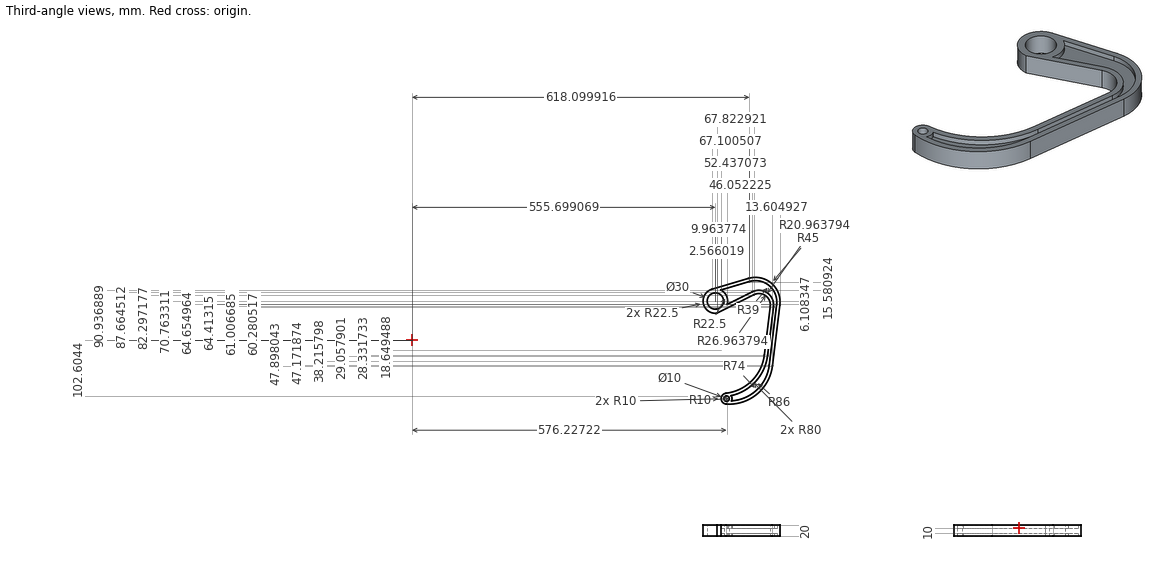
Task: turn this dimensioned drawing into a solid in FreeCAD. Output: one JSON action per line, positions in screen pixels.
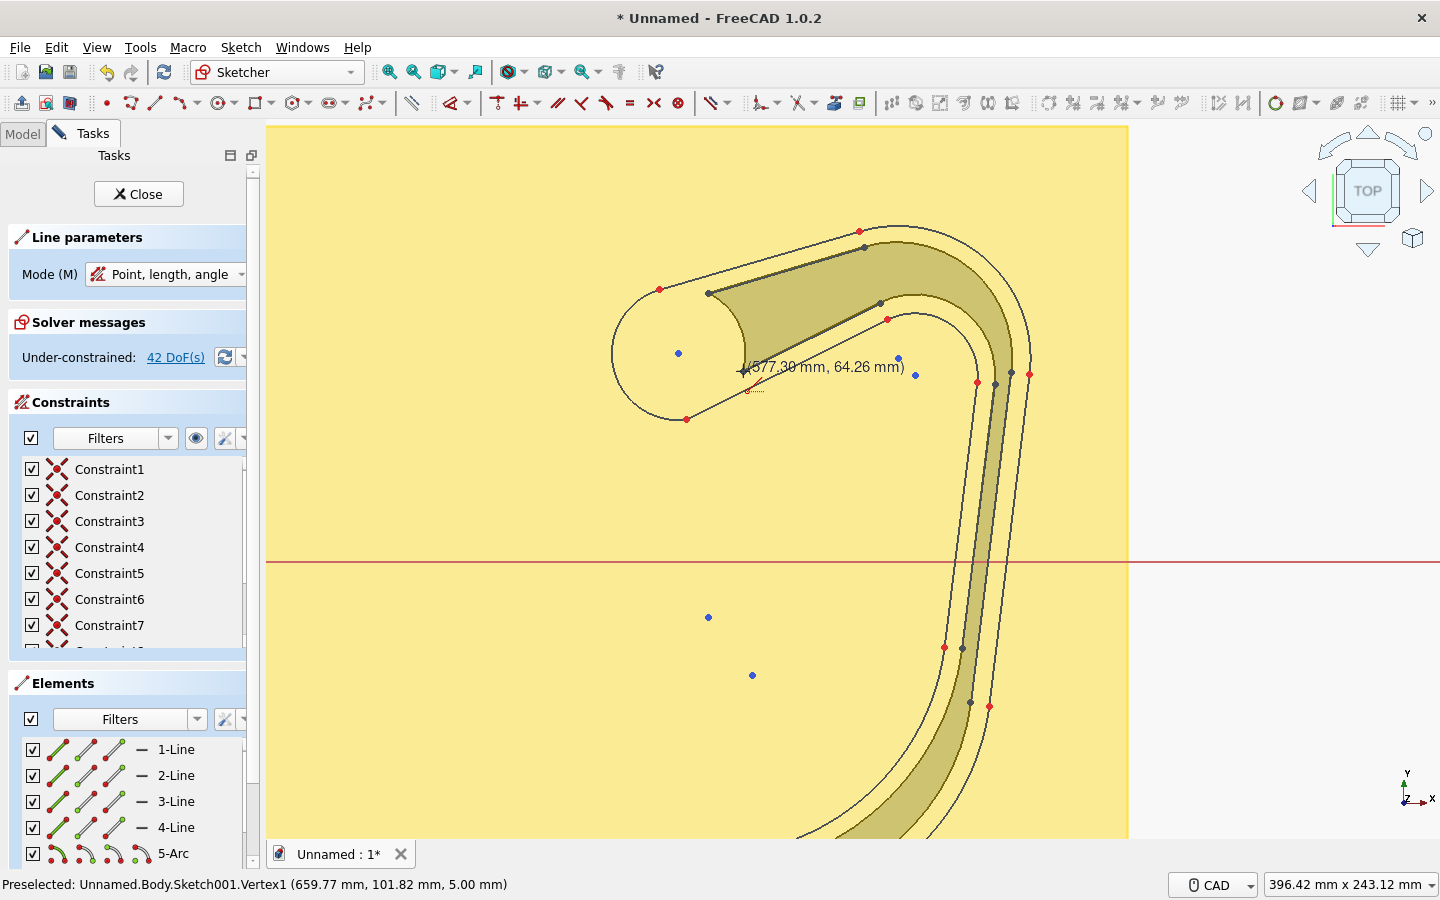
{"action": "left_click", "coordinate": [180, 104]}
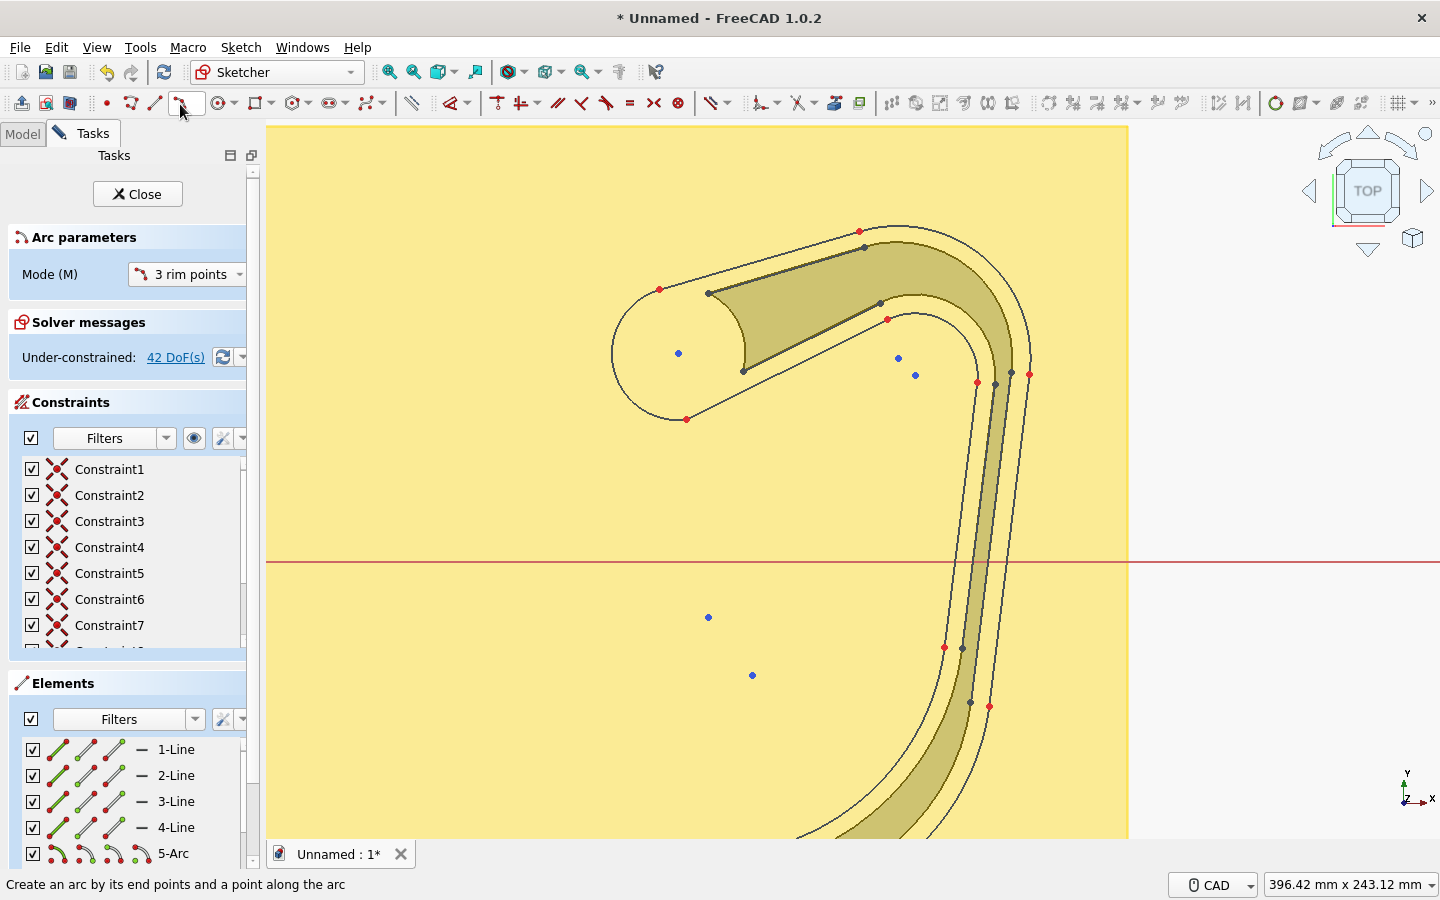
{"action": "left_click", "coordinate": [864, 248]}
{"action": "left_click", "coordinate": [1011, 373]}
{"action": "left_click", "coordinate": [1000, 305]}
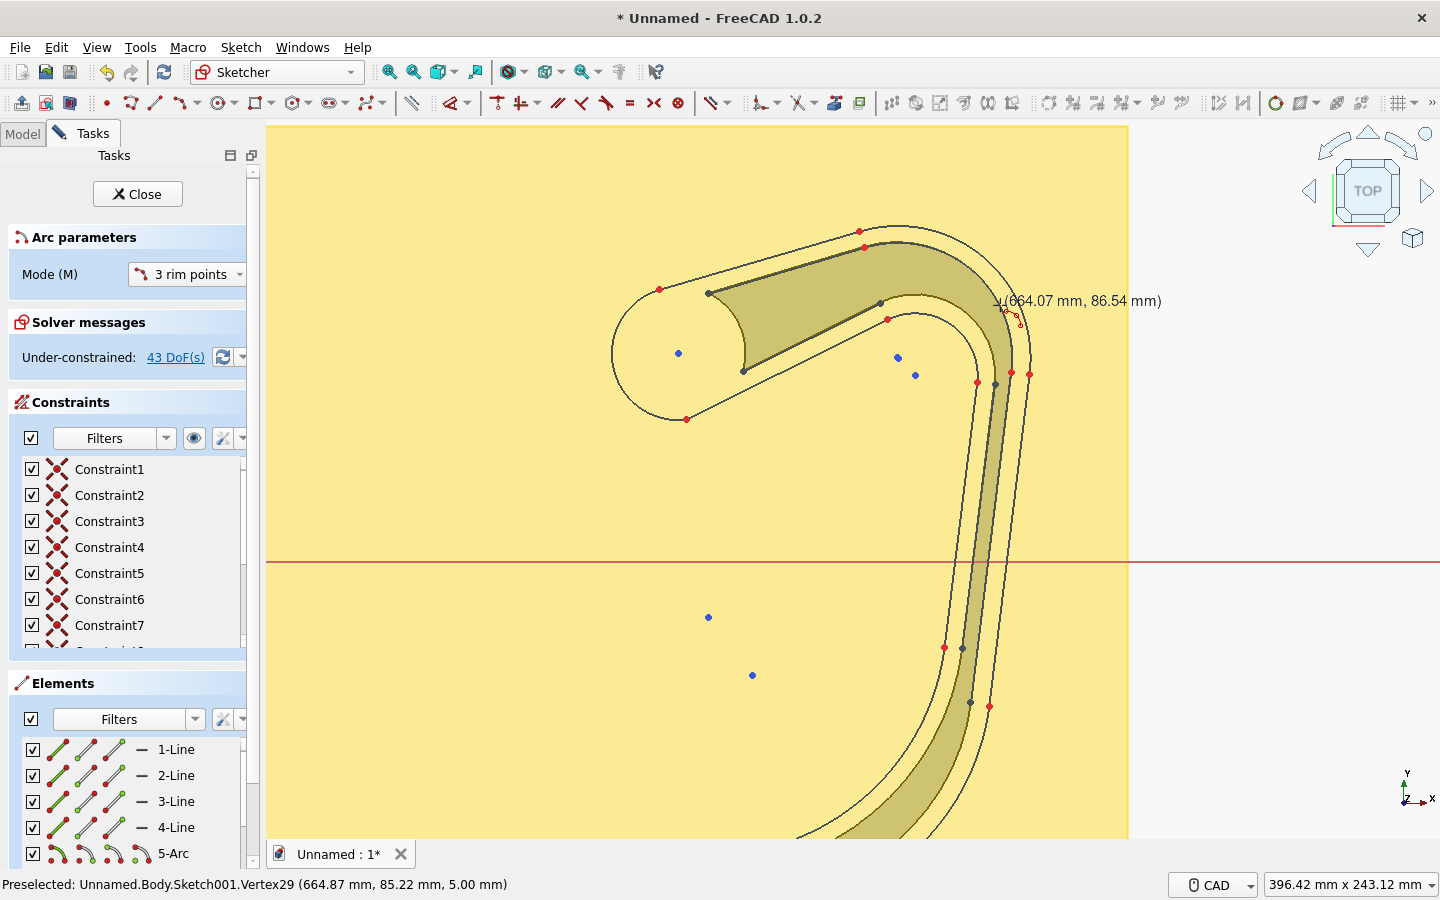
{"action": "left_click", "coordinate": [971, 703]}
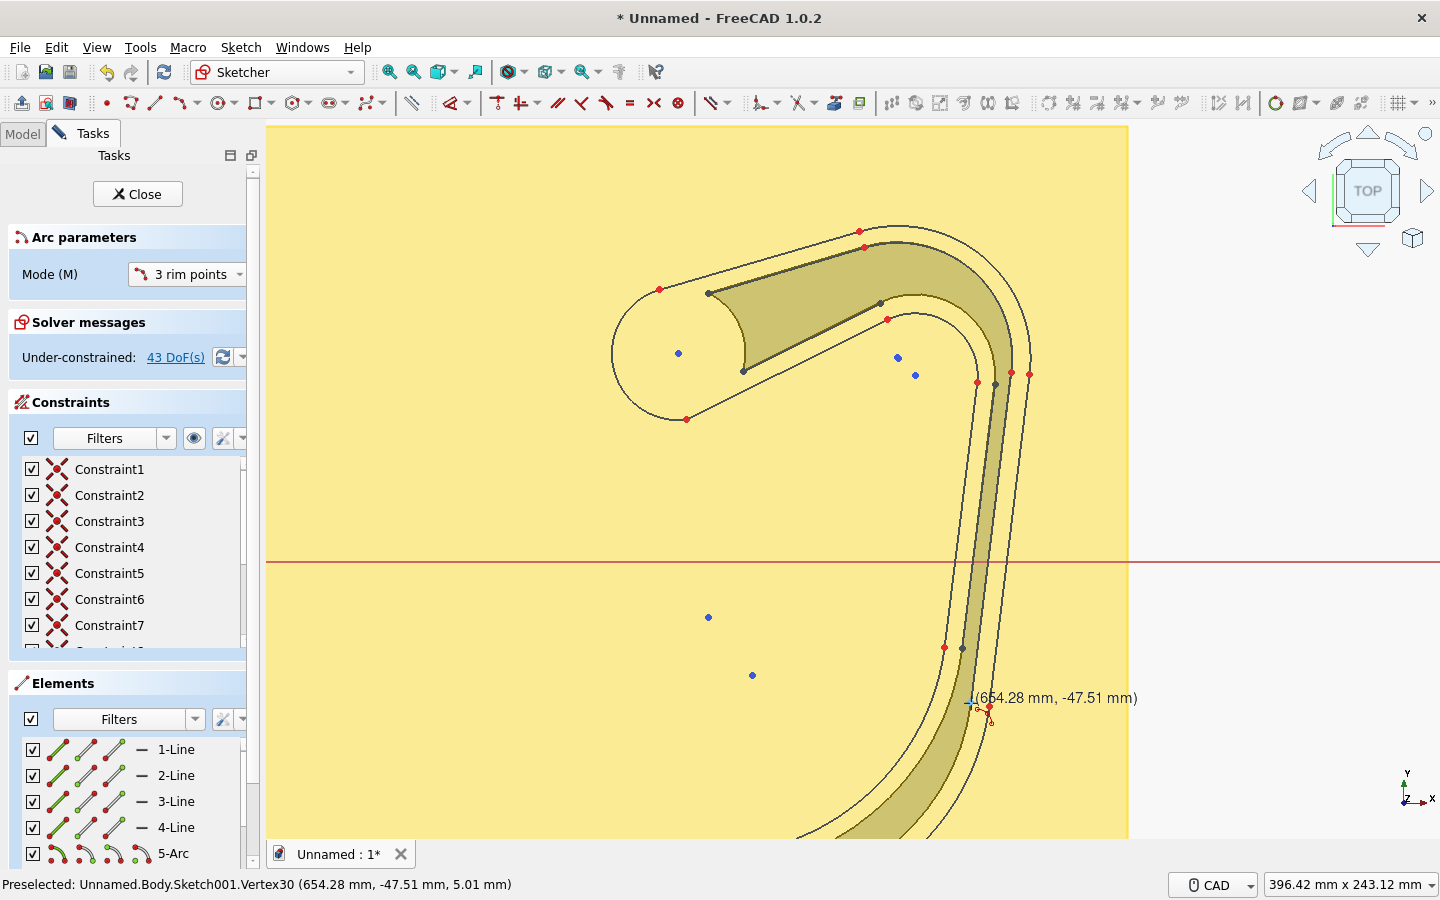
{"action": "scroll", "coordinate": [709, 292], "scroll_direction": "down", "scroll_amount": 2}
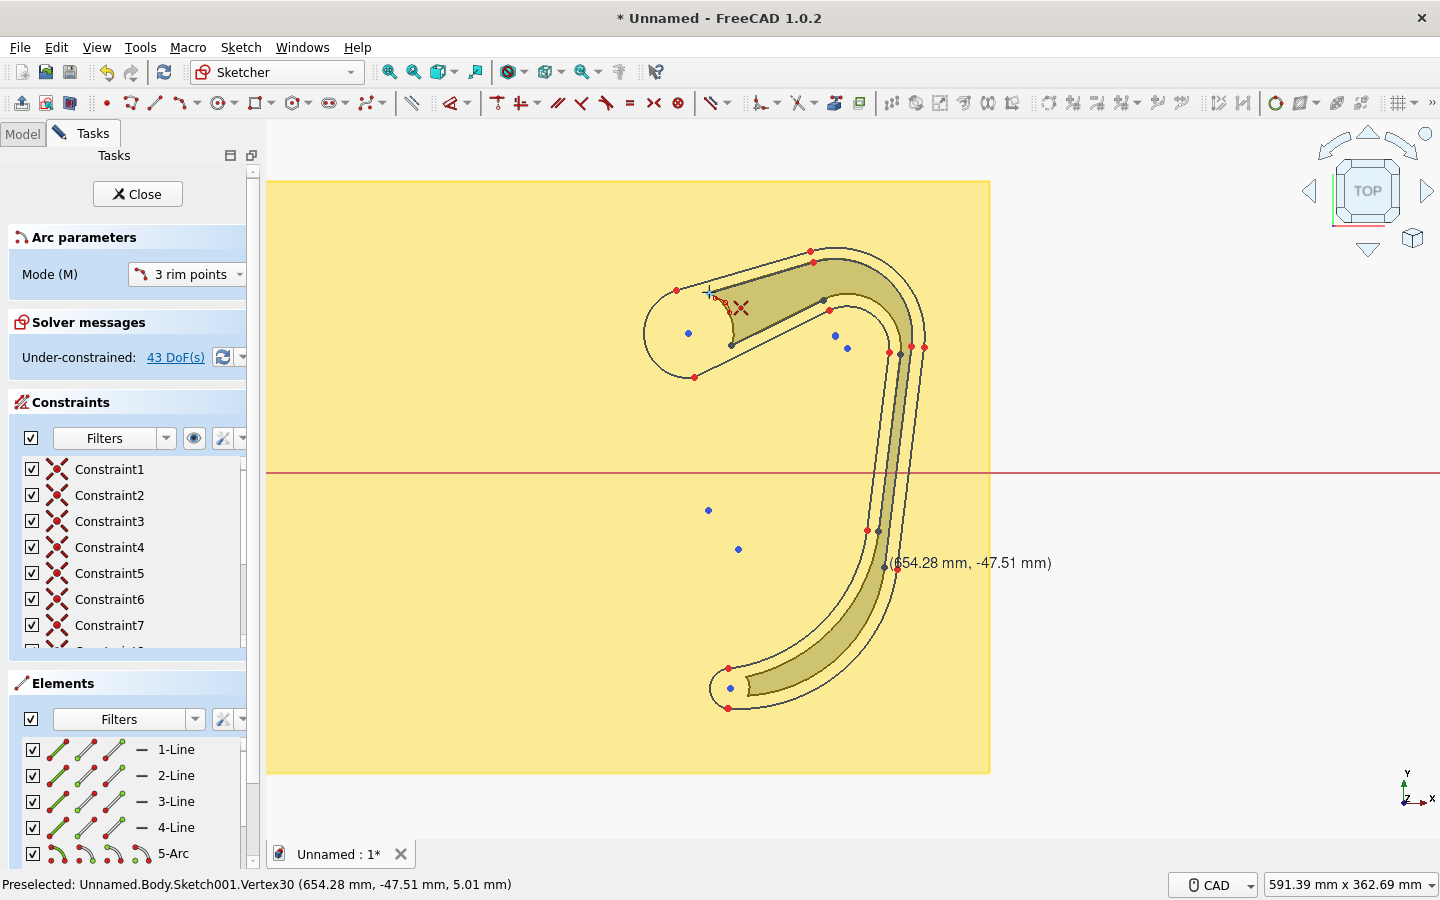
{"action": "scroll", "coordinate": [748, 696], "scroll_direction": "up", "scroll_amount": 2}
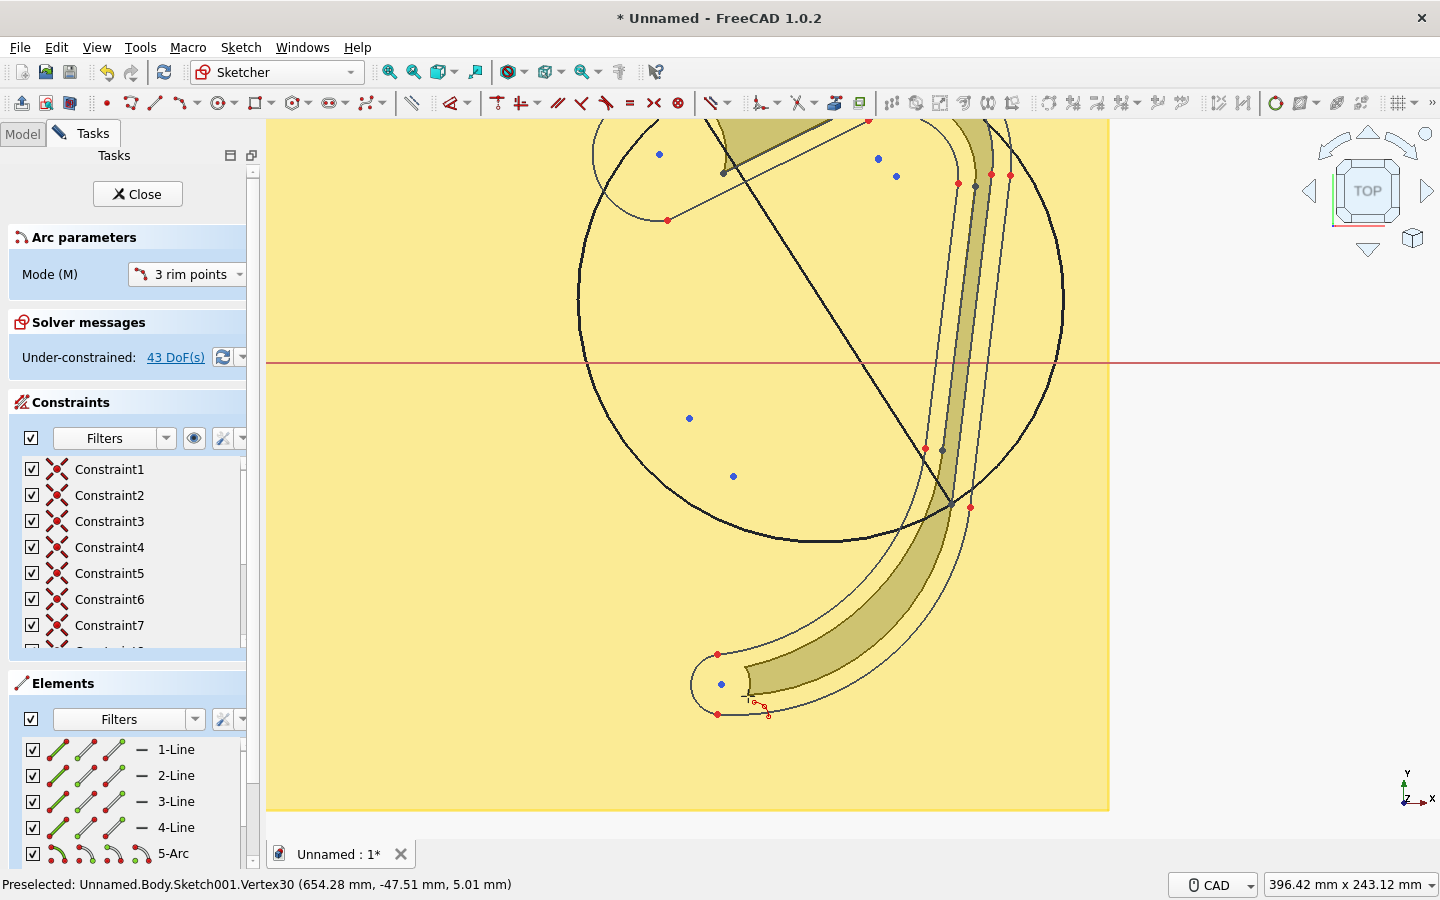
{"action": "left_click", "coordinate": [748, 695]}
{"action": "left_click", "coordinate": [861, 655]}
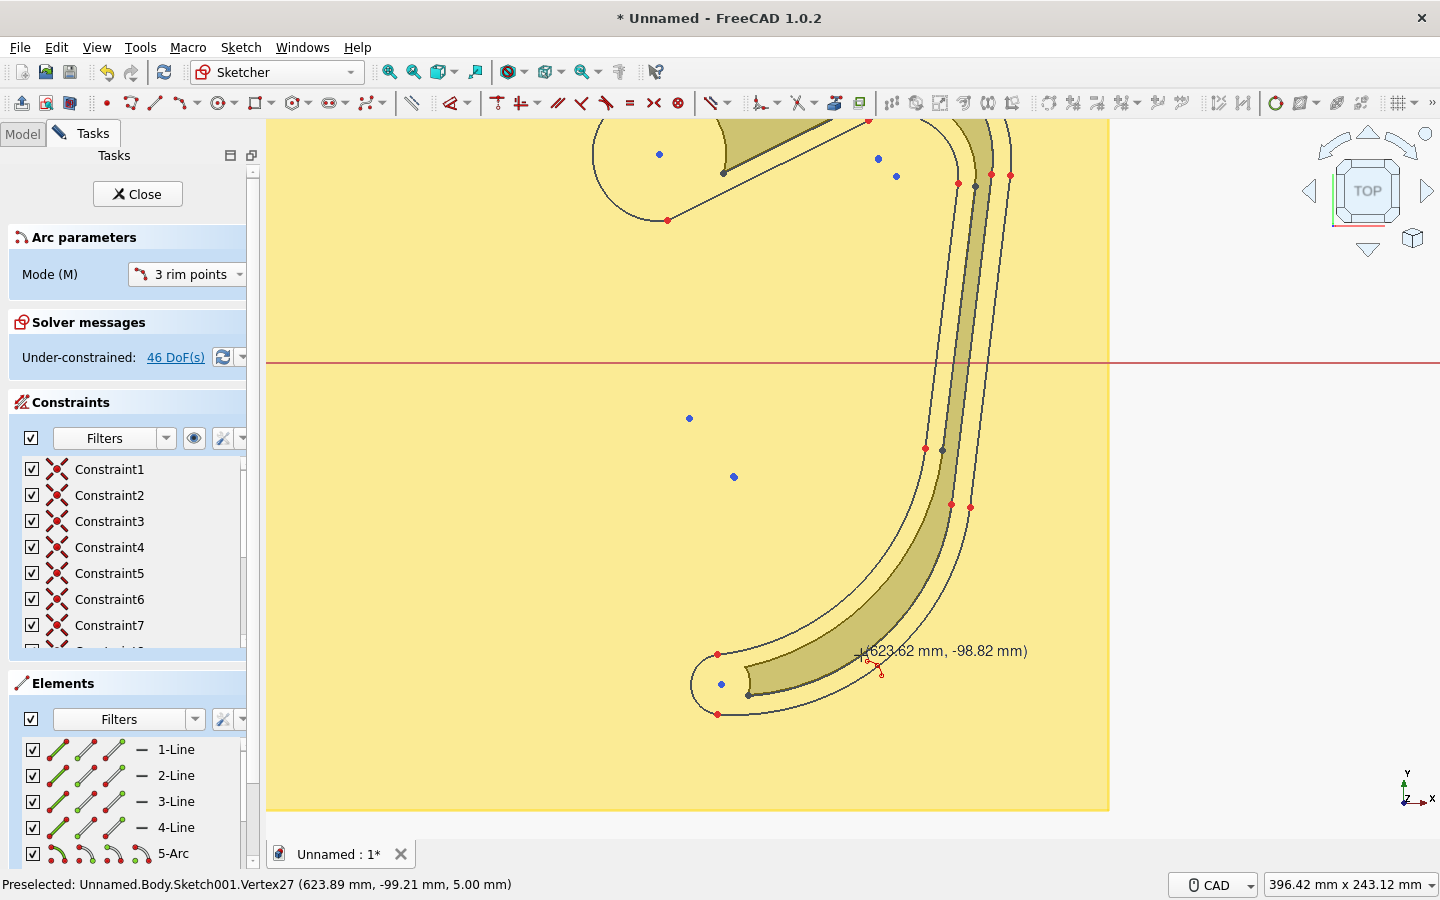
{"action": "left_click", "coordinate": [748, 696]}
{"action": "left_click", "coordinate": [745, 667]}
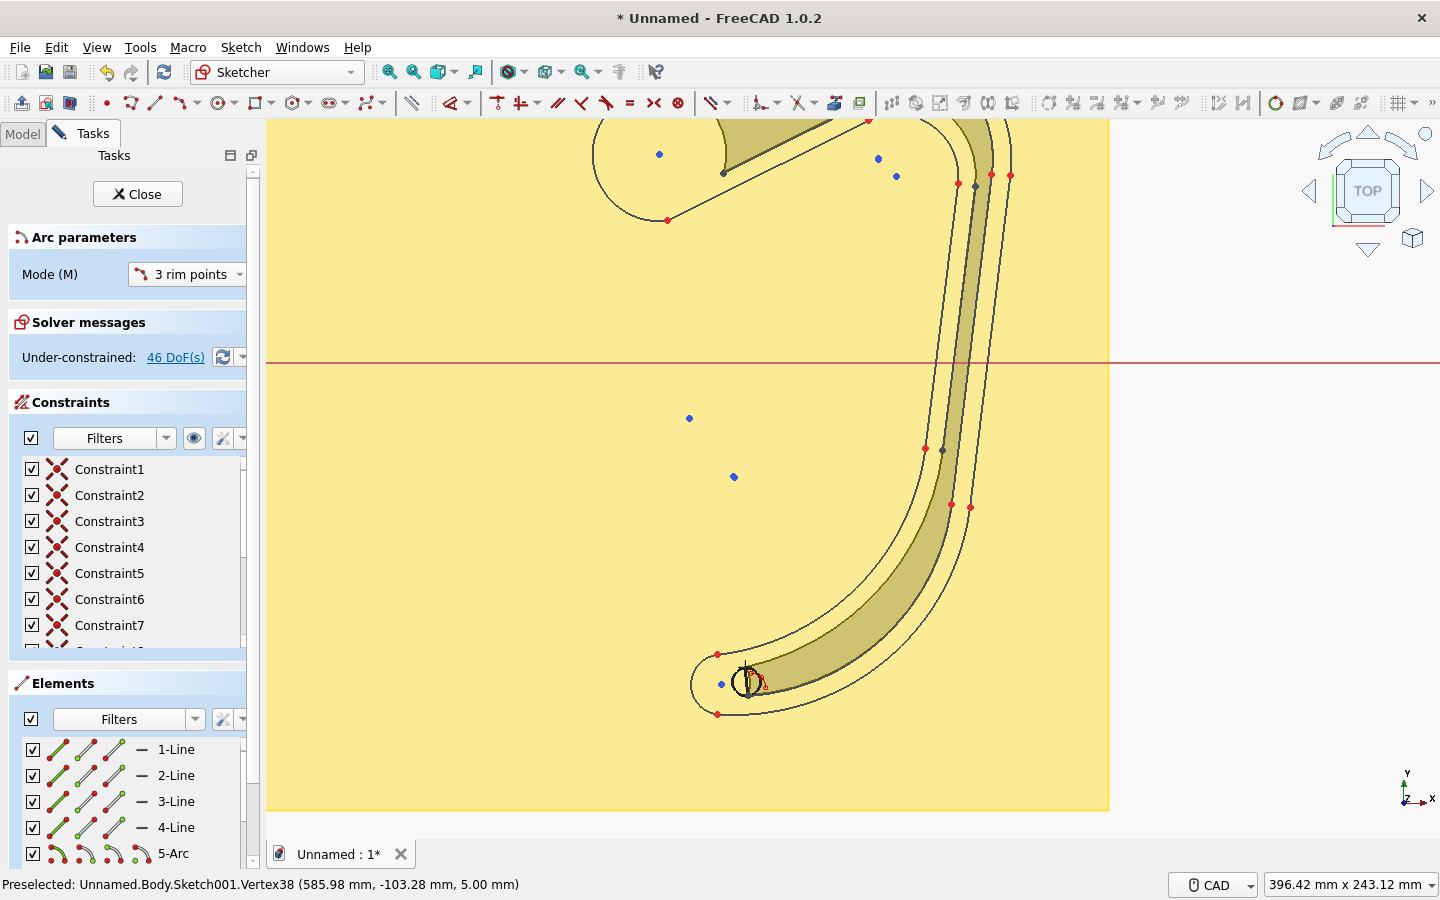
{"action": "scroll", "coordinate": [750, 681], "scroll_direction": "up", "scroll_amount": 8}